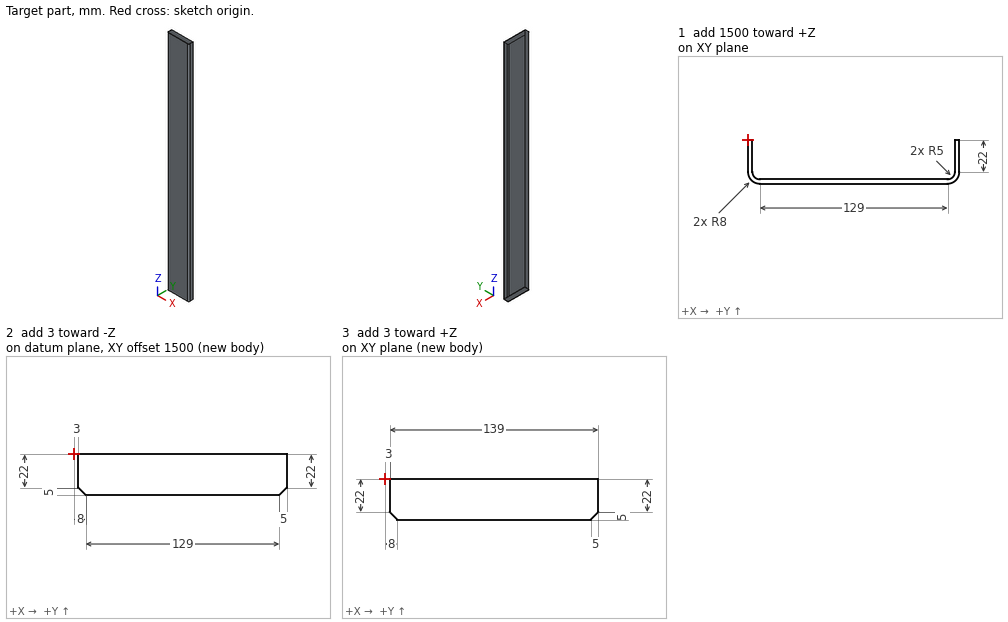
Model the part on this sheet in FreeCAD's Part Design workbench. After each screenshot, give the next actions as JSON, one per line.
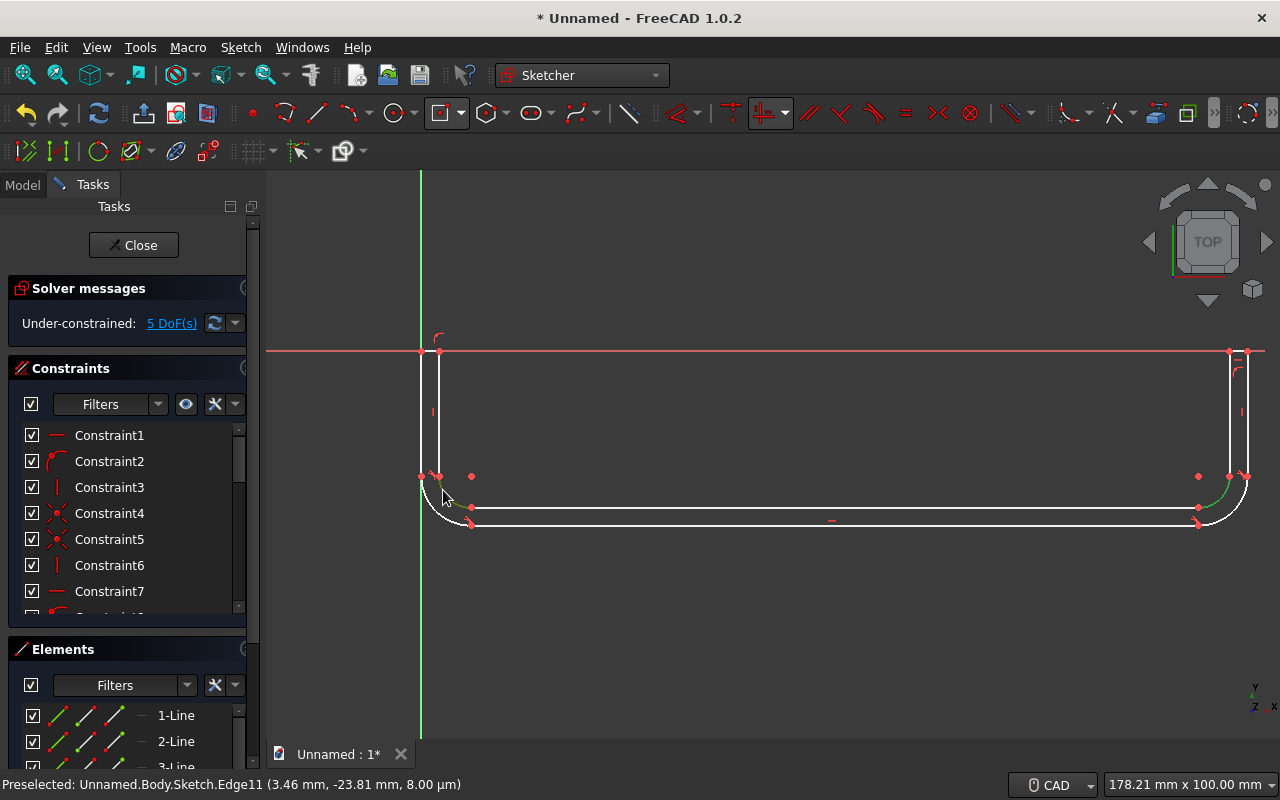
{"action": "key", "text": "e"}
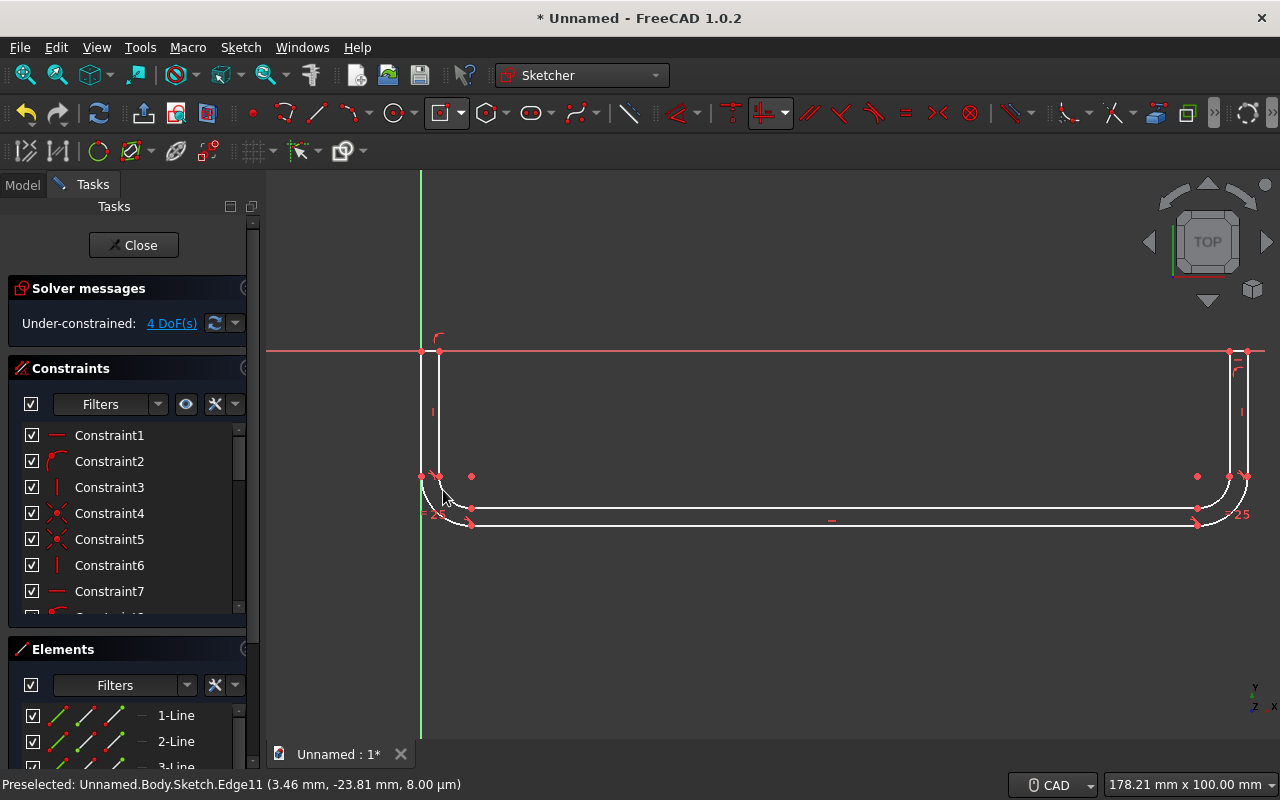
{"action": "scroll", "coordinate": [441, 491], "scroll_direction": "down", "scroll_amount": 2}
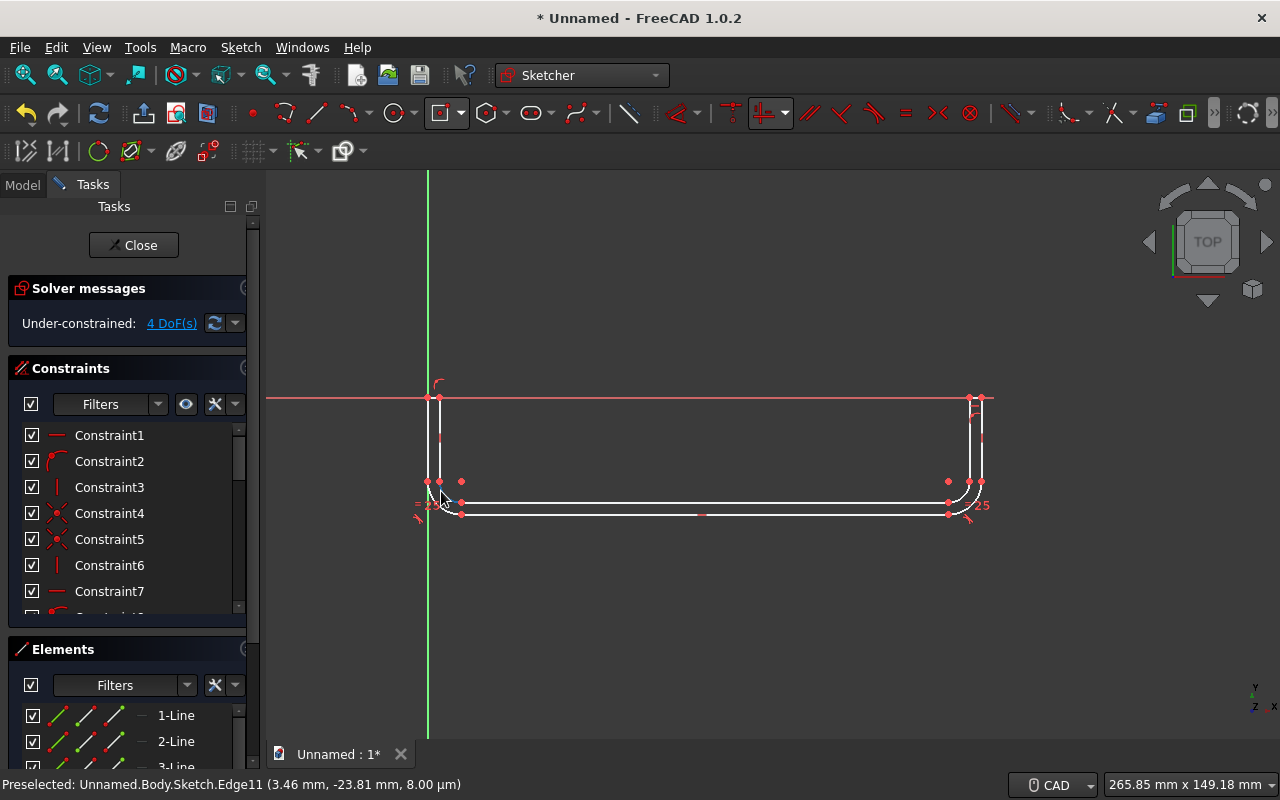
{"action": "scroll", "coordinate": [964, 511], "scroll_direction": "up", "scroll_amount": 2}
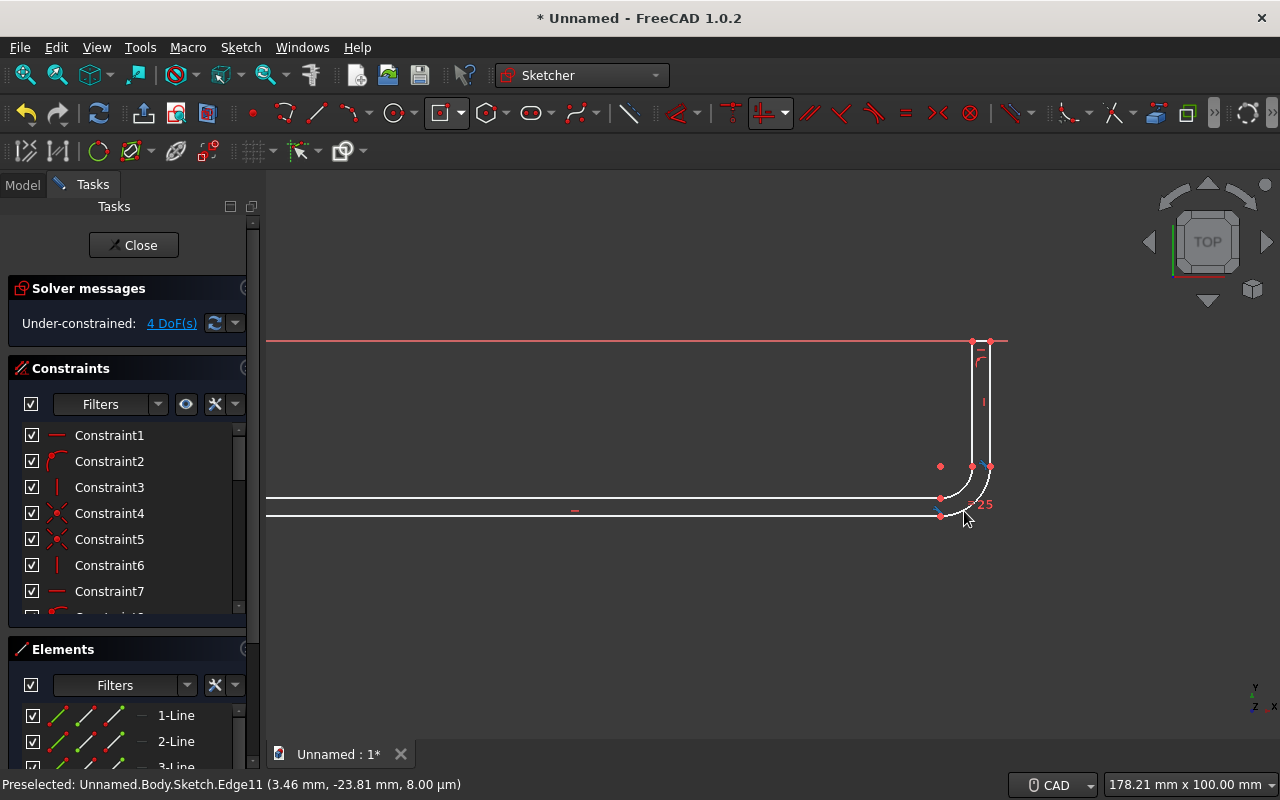
{"action": "left_click", "coordinate": [963, 511]}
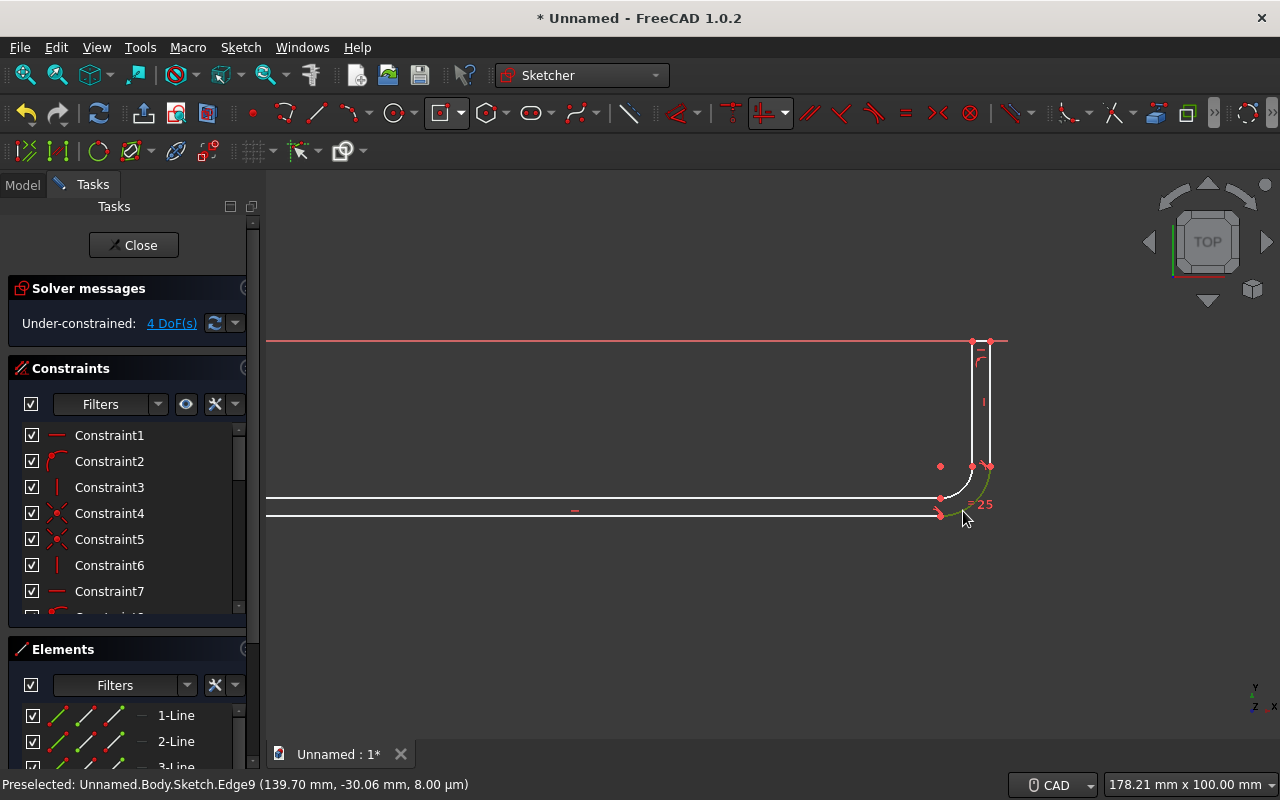
{"action": "key", "text": "k r"}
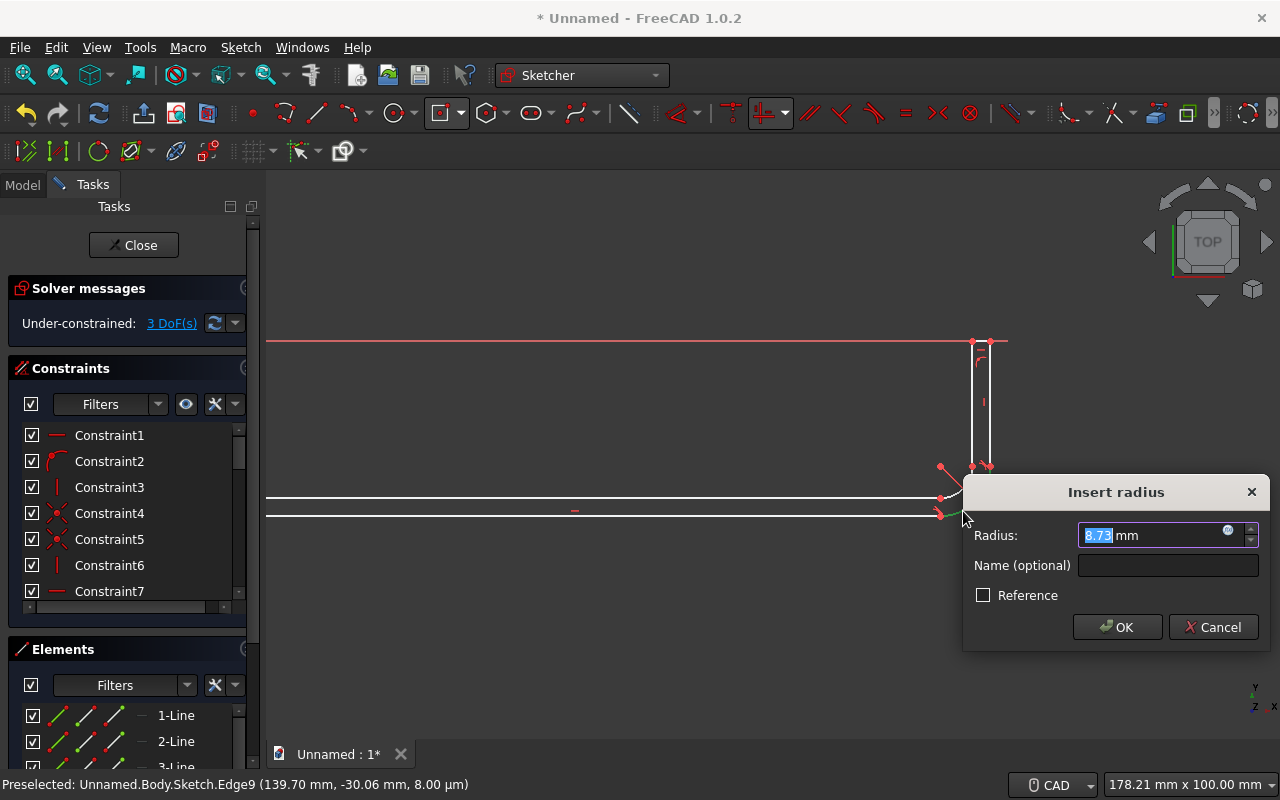
{"action": "type", "text": "8"}
{"action": "key", "text": "Return"}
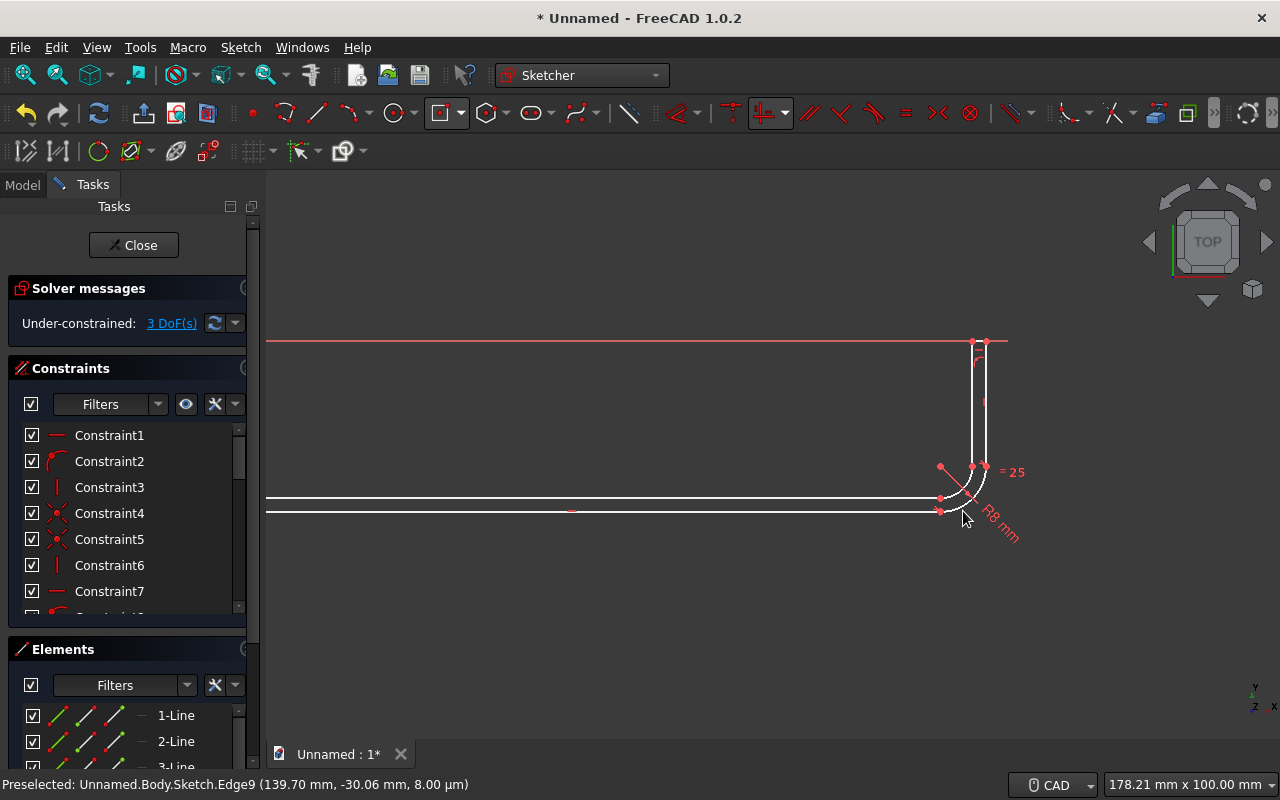
{"action": "scroll", "coordinate": [955, 495], "scroll_direction": "up", "scroll_amount": 2}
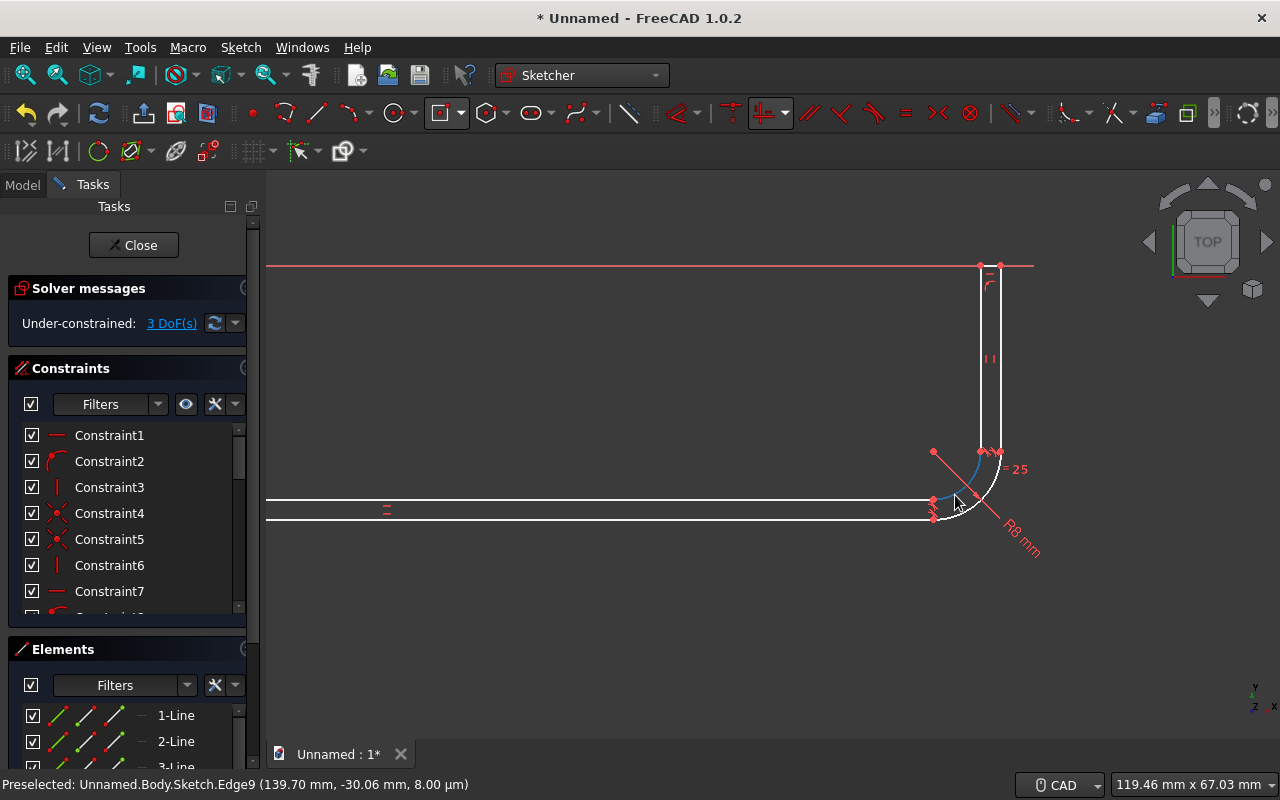
{"action": "left_click", "coordinate": [955, 494]}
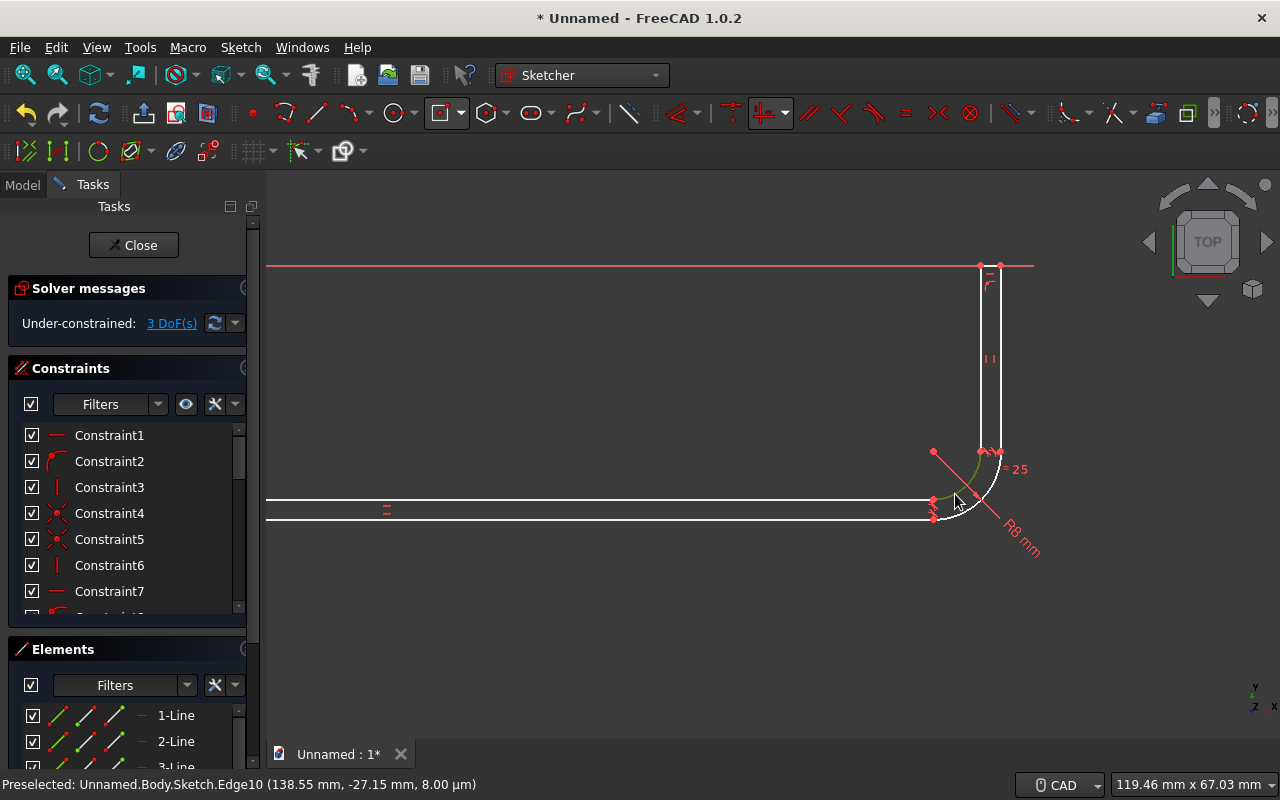
{"action": "left_click", "coordinate": [700, 114]}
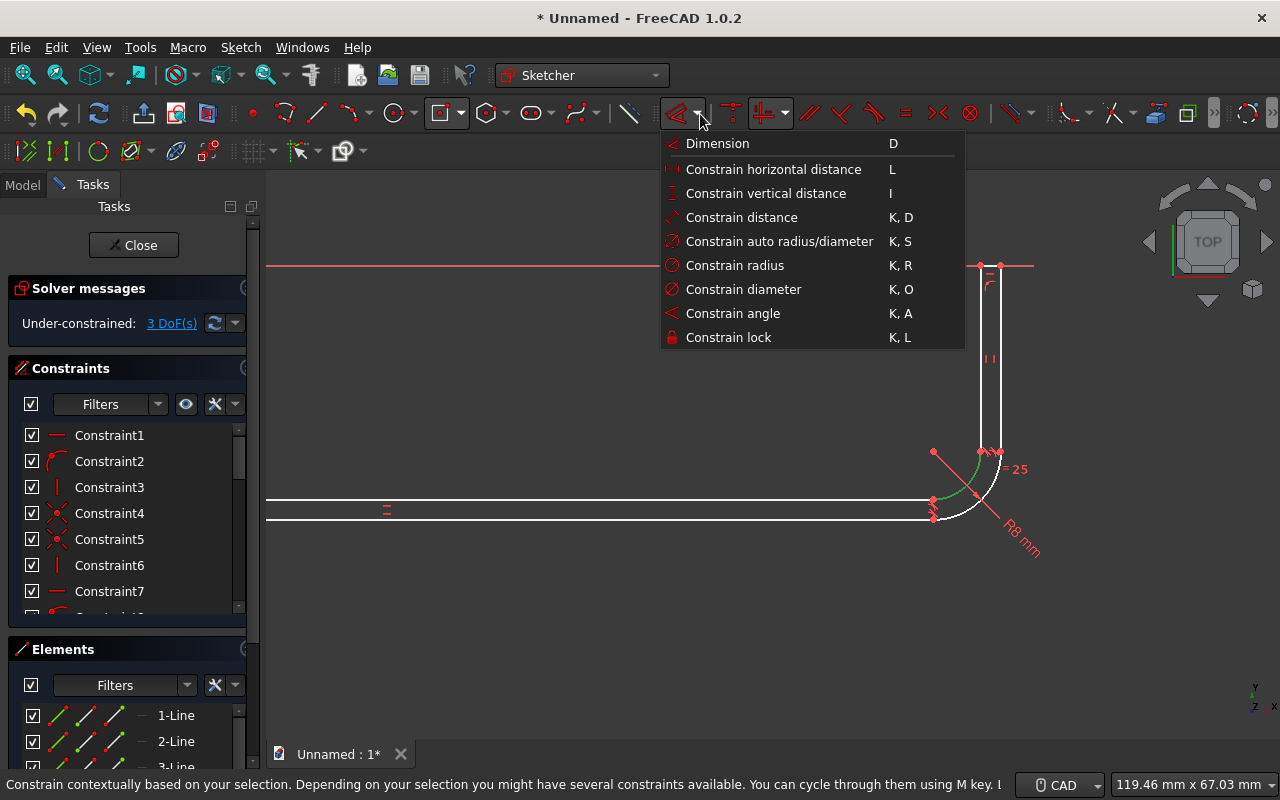
{"action": "left_click", "coordinate": [813, 265]}